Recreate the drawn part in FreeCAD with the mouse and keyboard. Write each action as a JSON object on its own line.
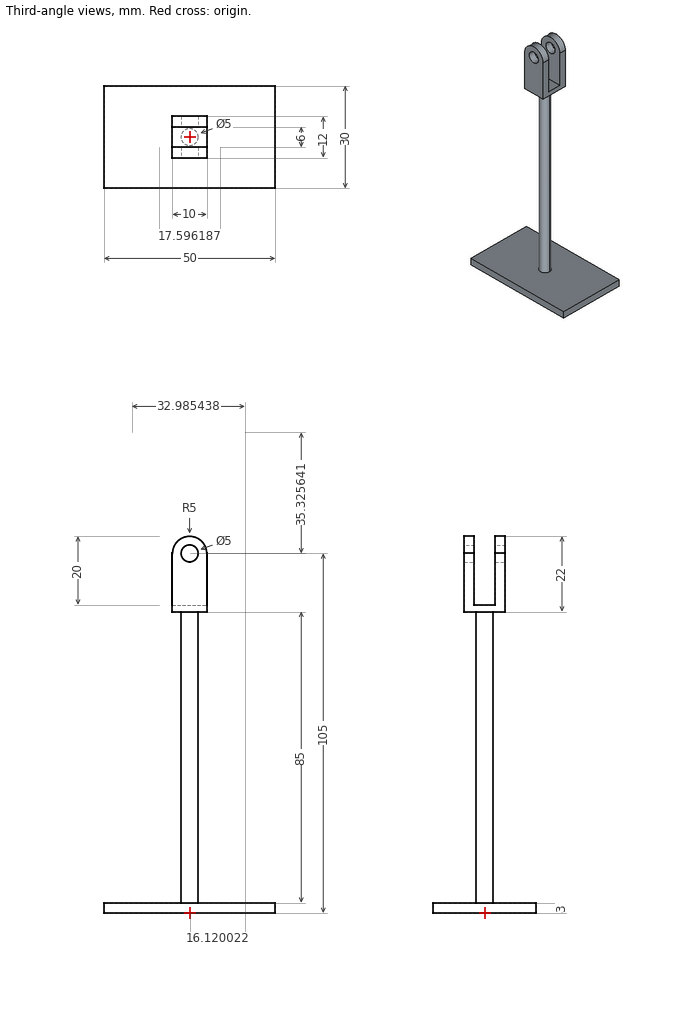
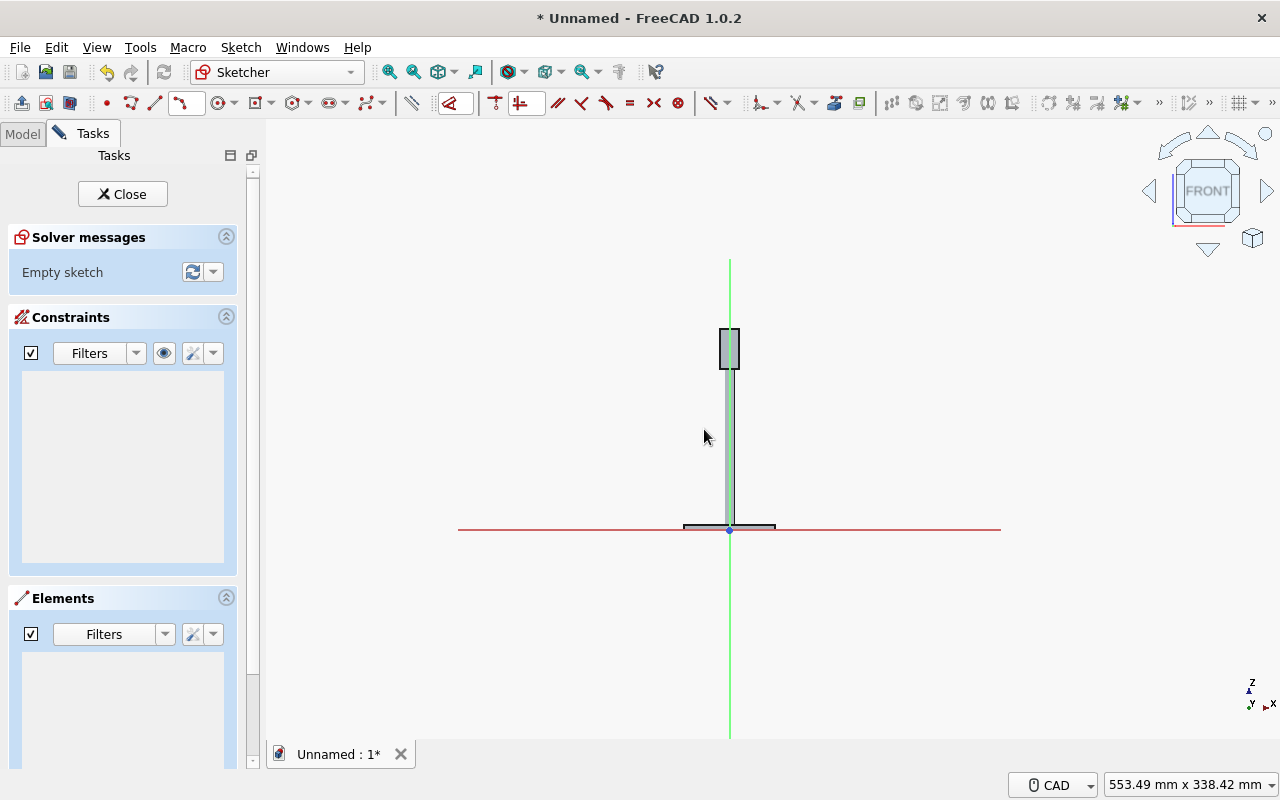
{"action": "scroll", "coordinate": [734, 284], "scroll_direction": "up", "scroll_amount": 9}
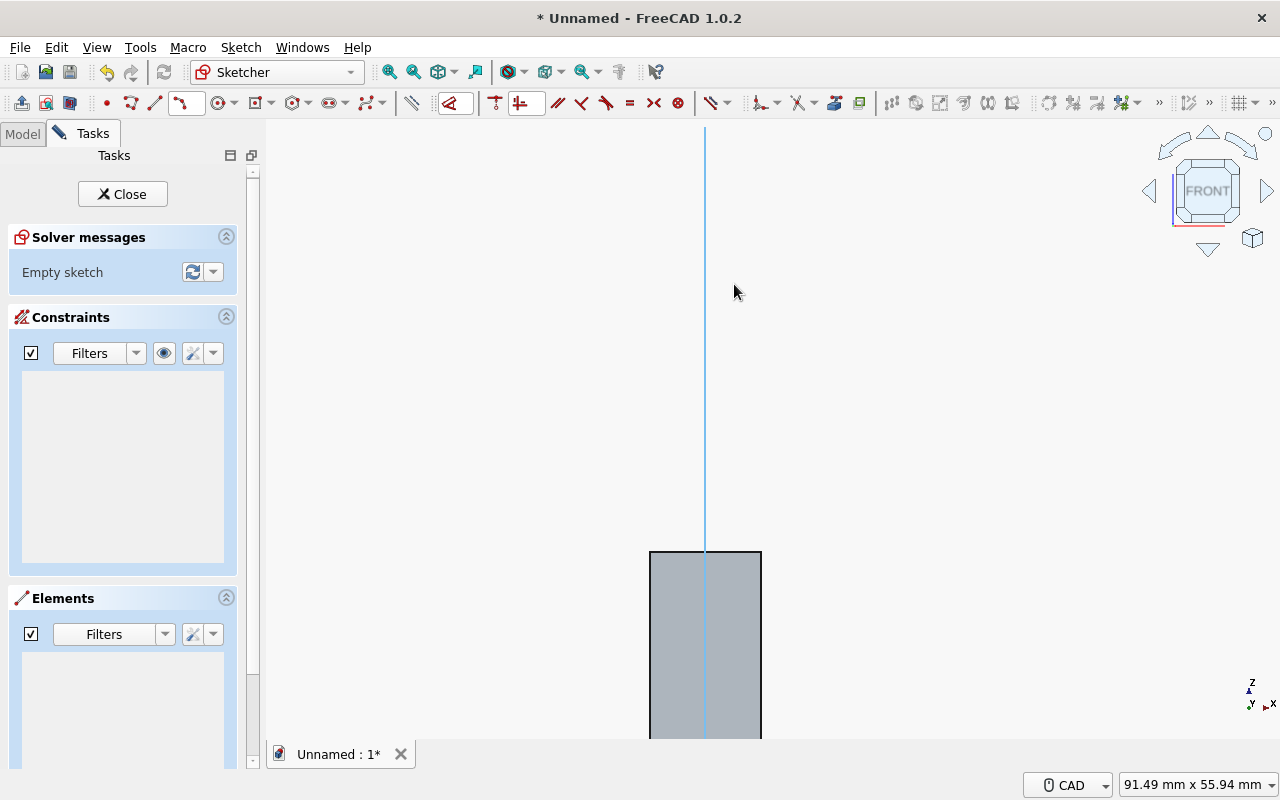
{"action": "left_click", "coordinate": [132, 104]}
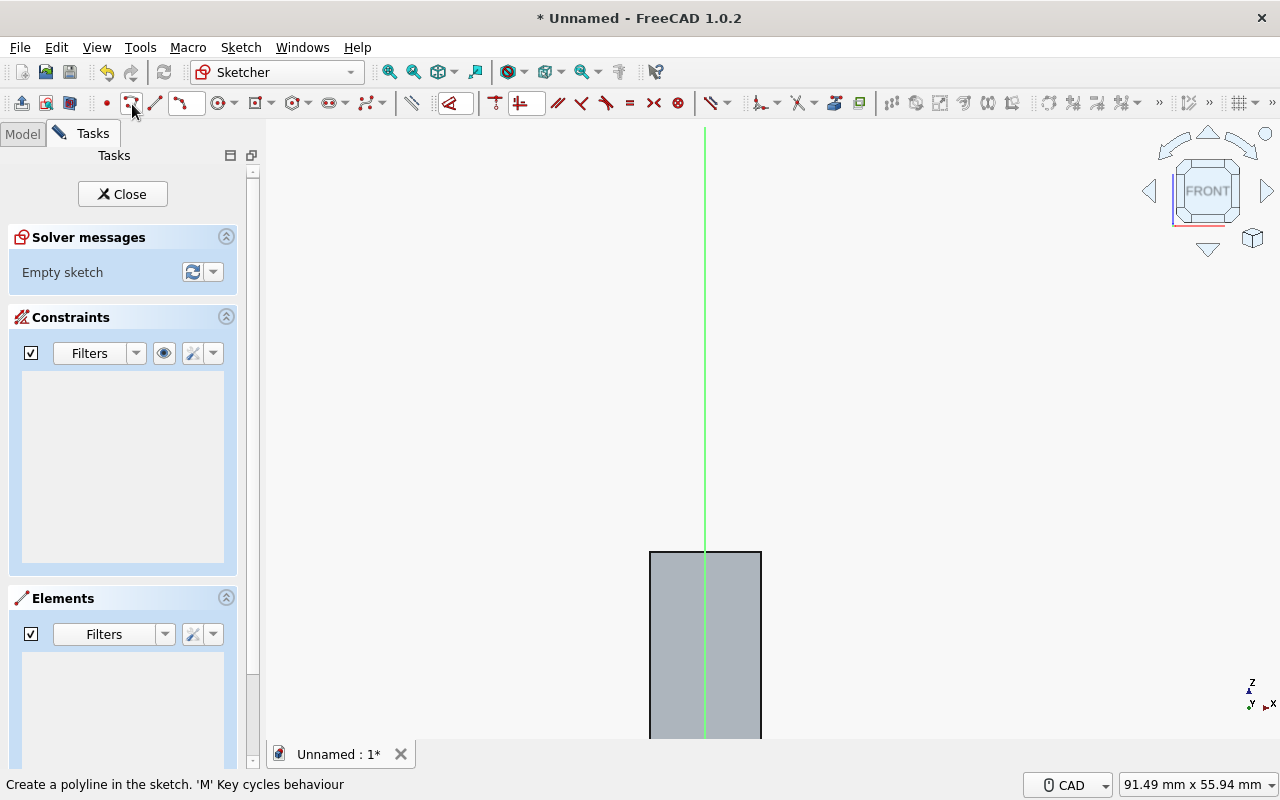
{"action": "left_click", "coordinate": [761, 608]}
{"action": "left_click", "coordinate": [884, 216]}
{"action": "left_click", "coordinate": [518, 216]}
{"action": "left_click", "coordinate": [650, 608]}
{"action": "right_click", "coordinate": [650, 608]}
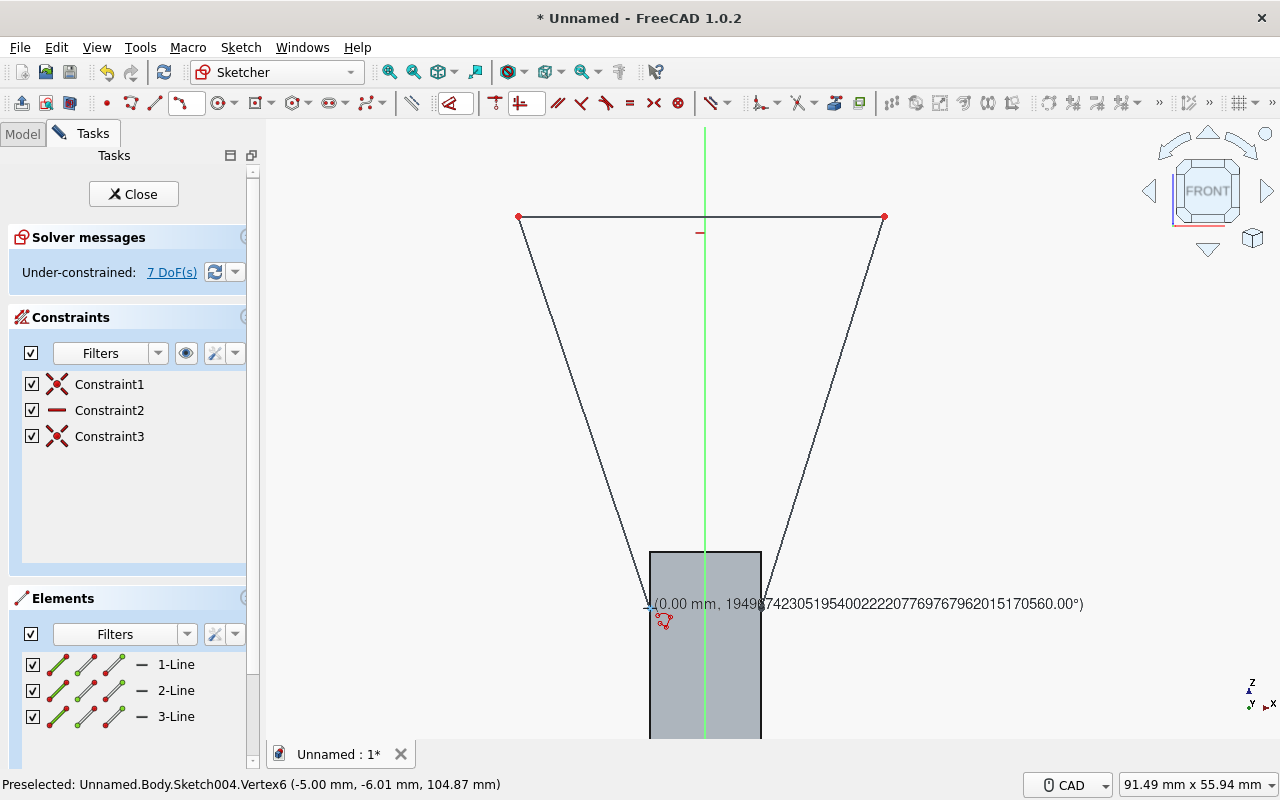
{"action": "left_click", "coordinate": [180, 104]}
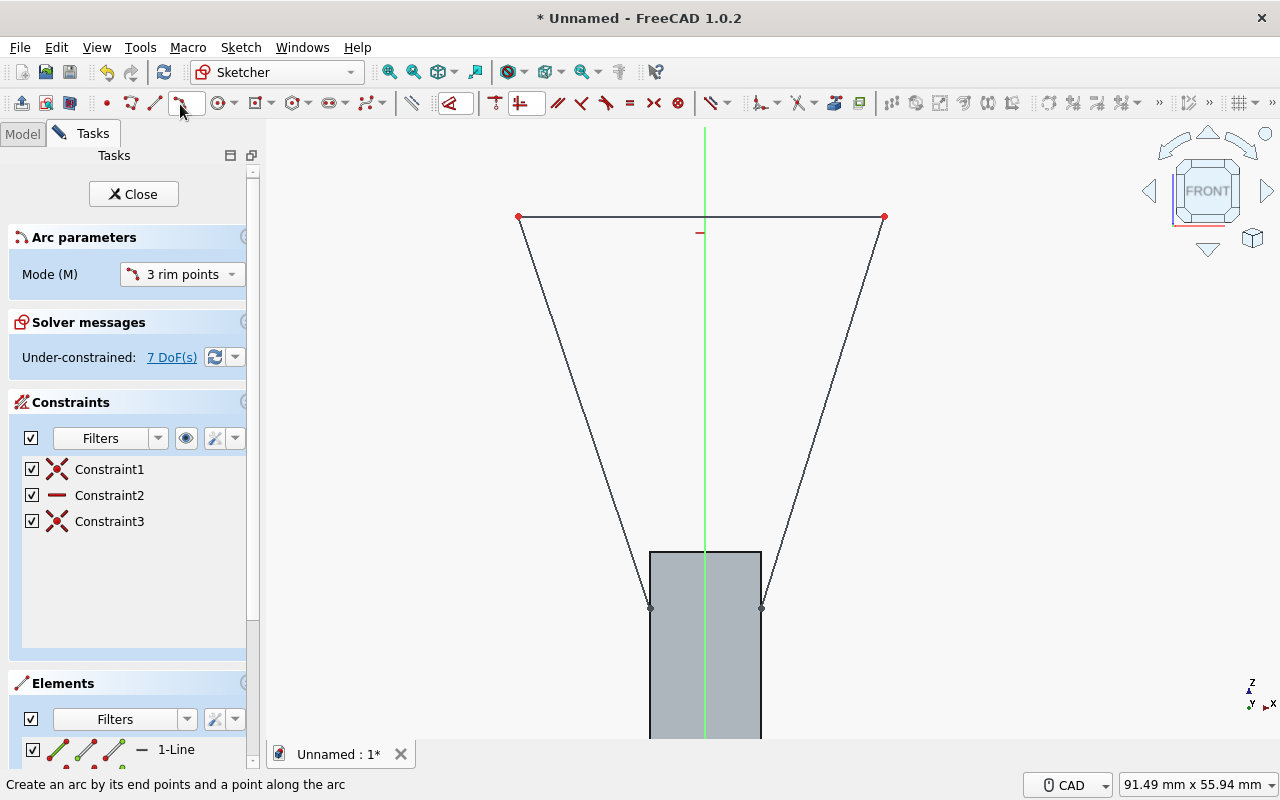
{"action": "left_click", "coordinate": [650, 609]}
{"action": "left_click", "coordinate": [761, 609]}
{"action": "left_click", "coordinate": [723, 555]}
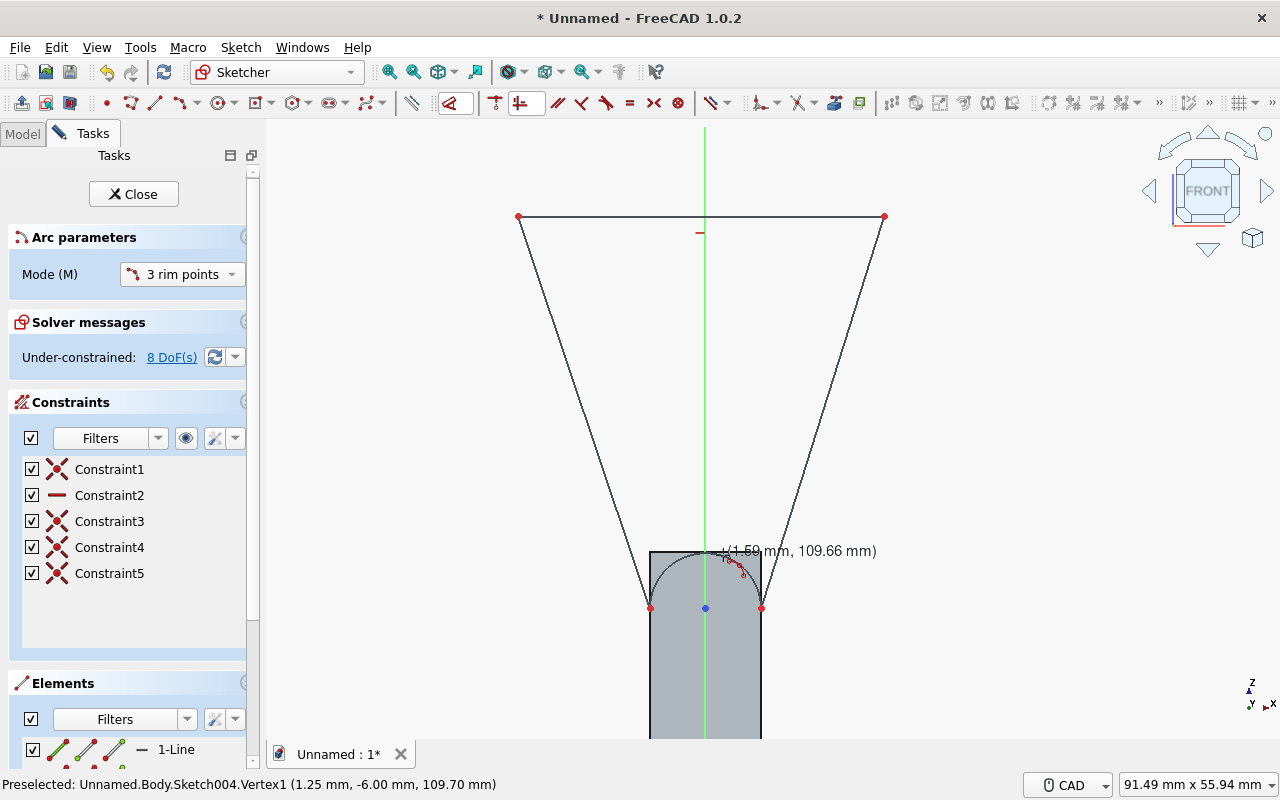
{"action": "left_click", "coordinate": [218, 104]}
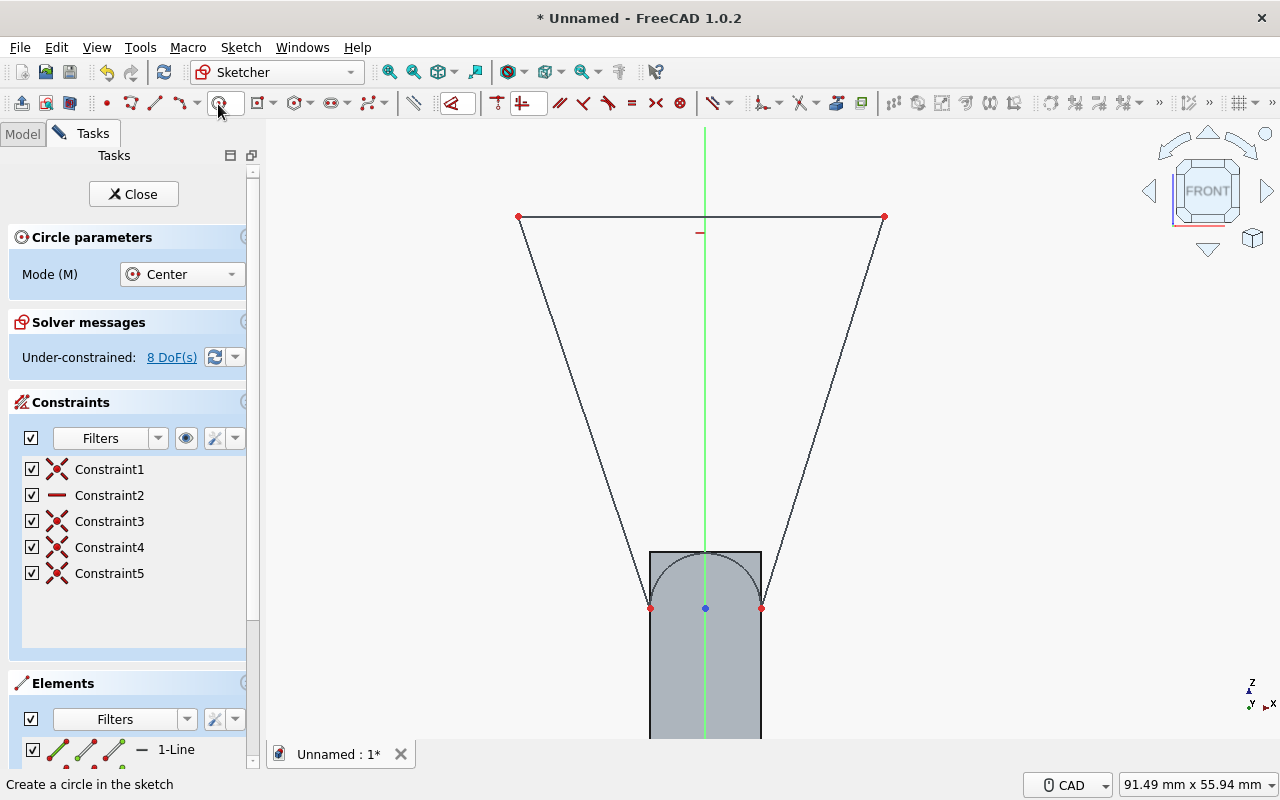
{"action": "left_click", "coordinate": [705, 608]}
{"action": "mouse_move", "coordinate": [725, 588]}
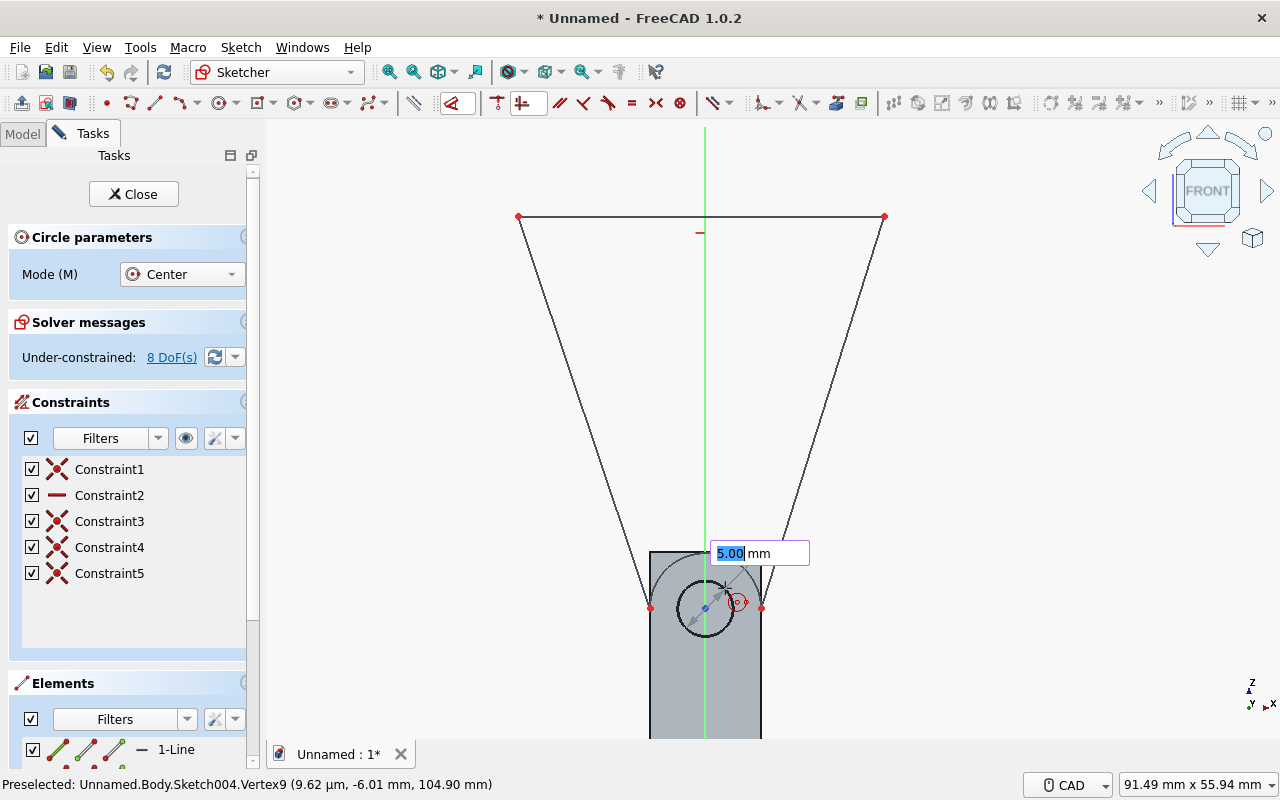
{"action": "type", "text": "5"}
{"action": "key", "text": "Return"}
{"action": "key", "text": "Escape"}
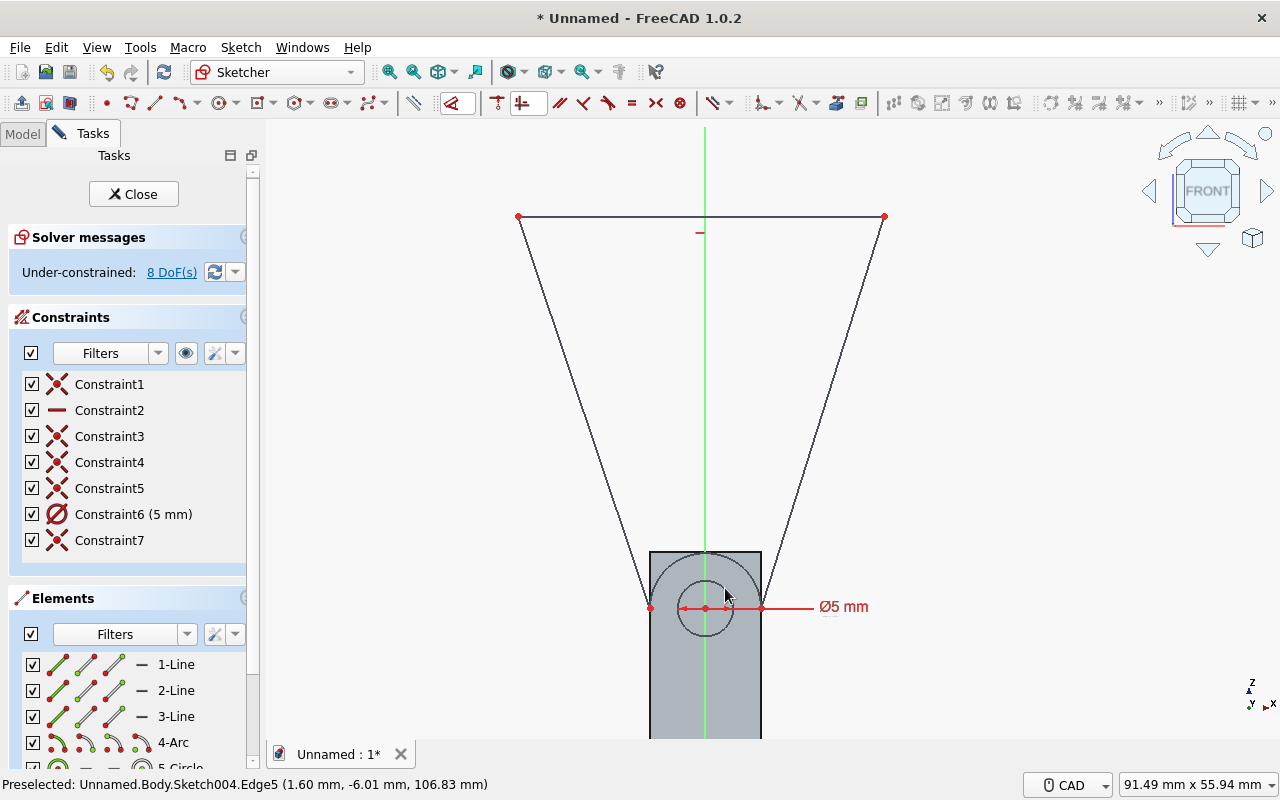
{"action": "left_click", "coordinate": [706, 609]}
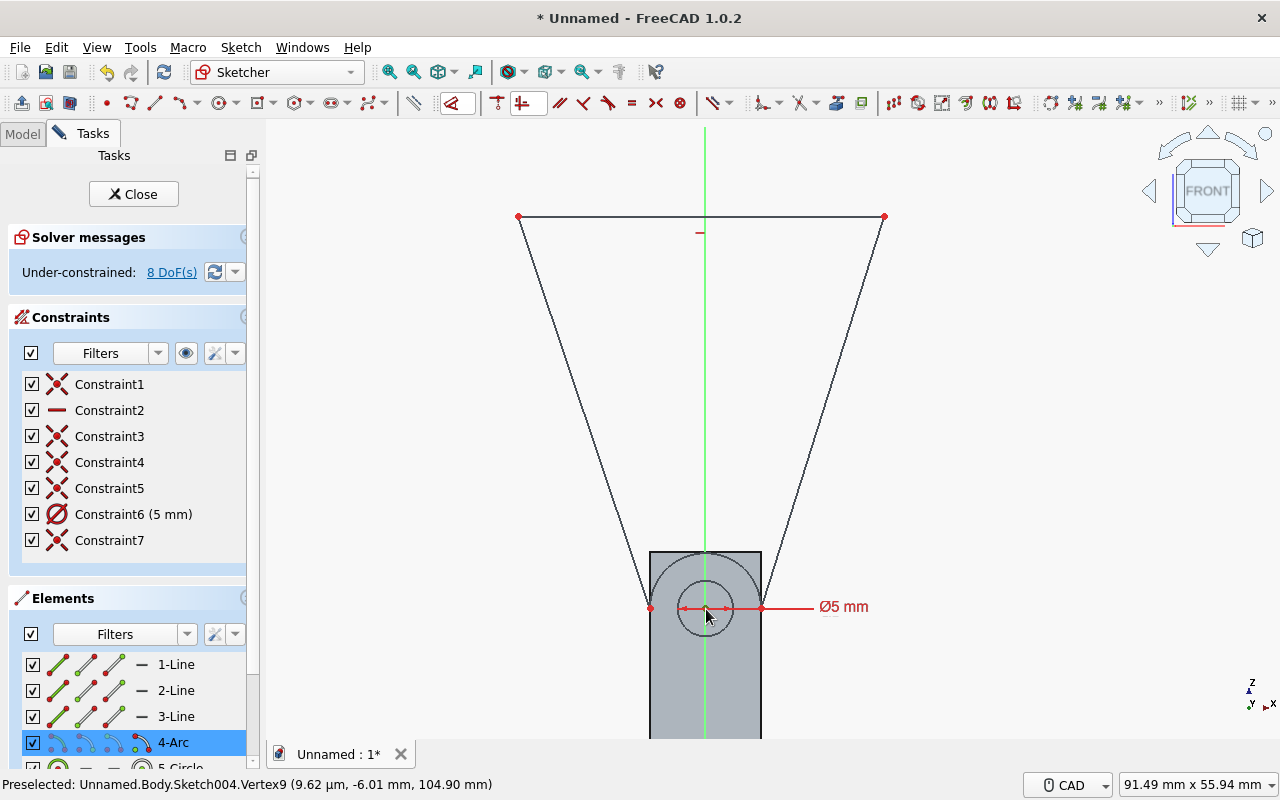
{"action": "left_click", "coordinate": [705, 671]}